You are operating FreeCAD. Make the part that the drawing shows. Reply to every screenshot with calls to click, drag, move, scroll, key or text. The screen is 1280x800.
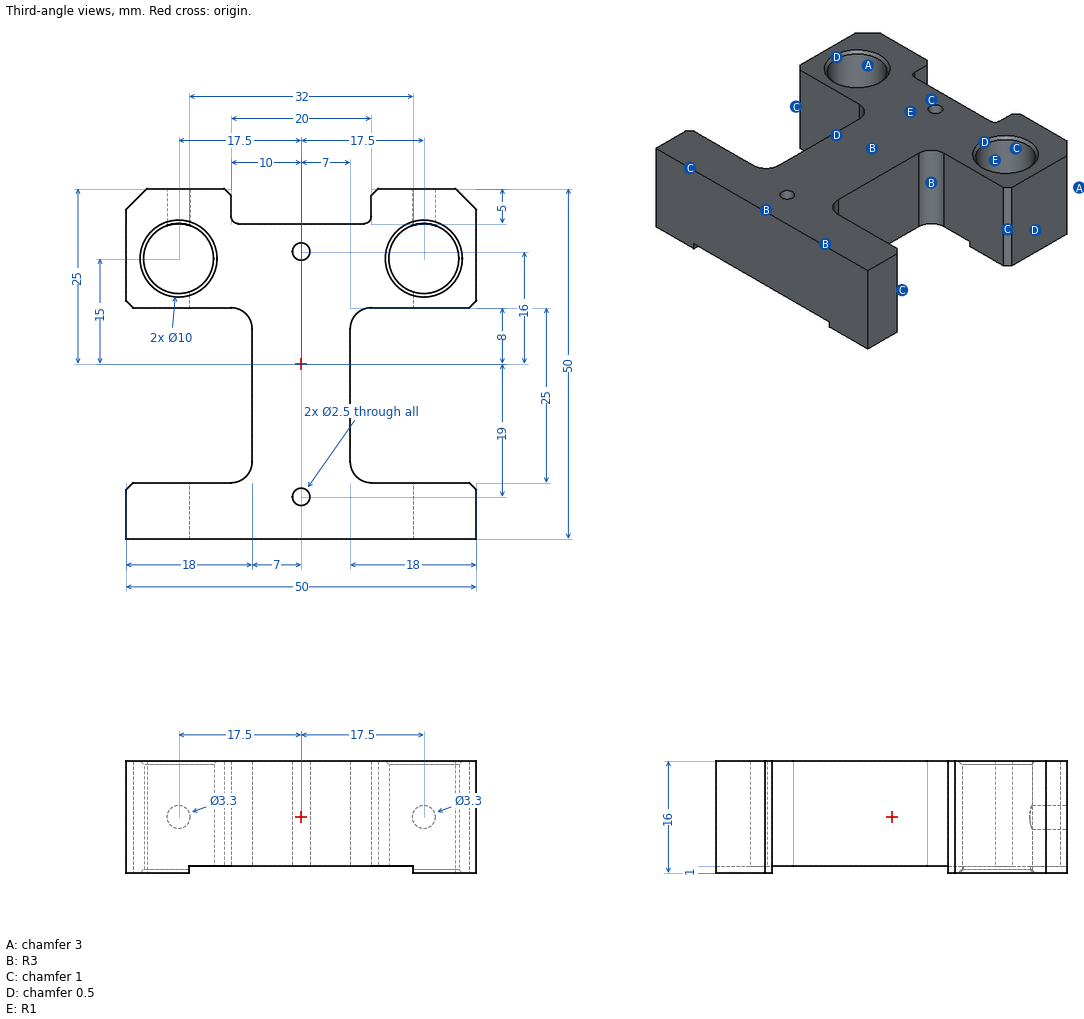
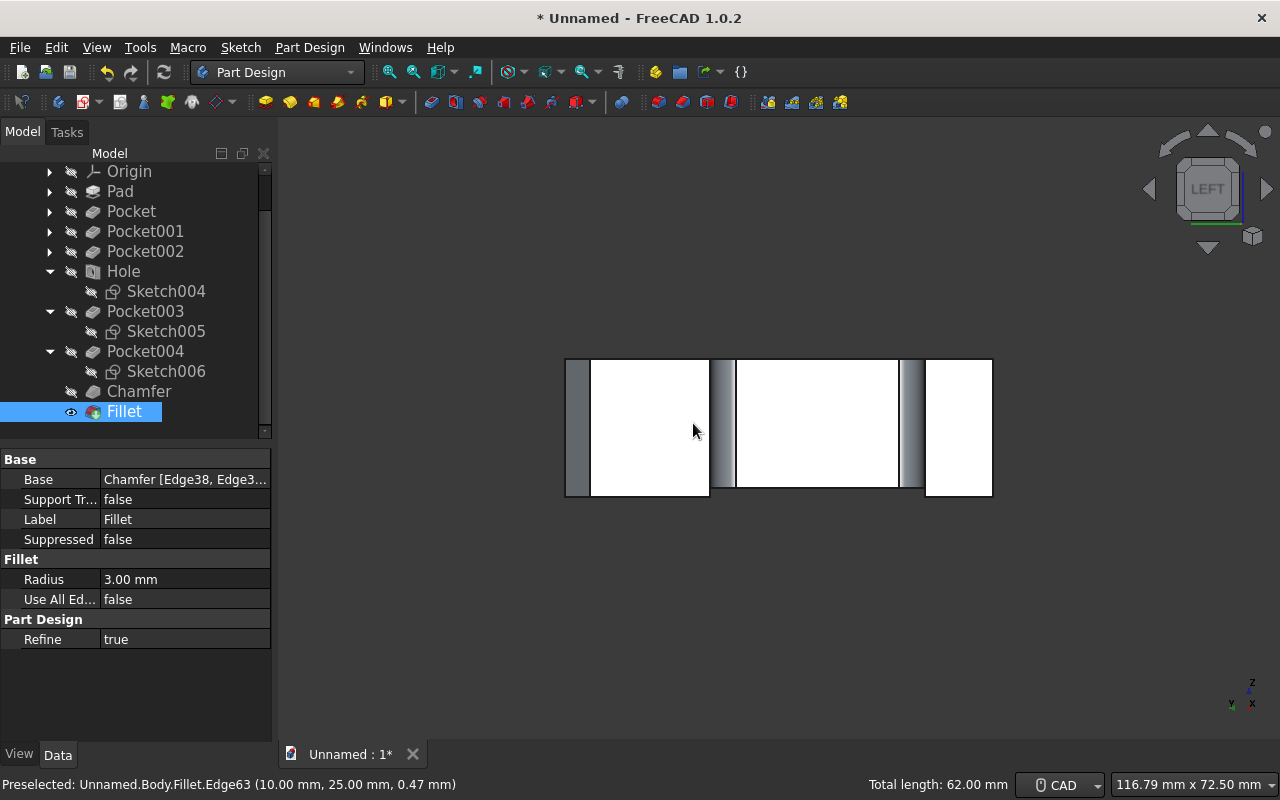
key(v)
key(f)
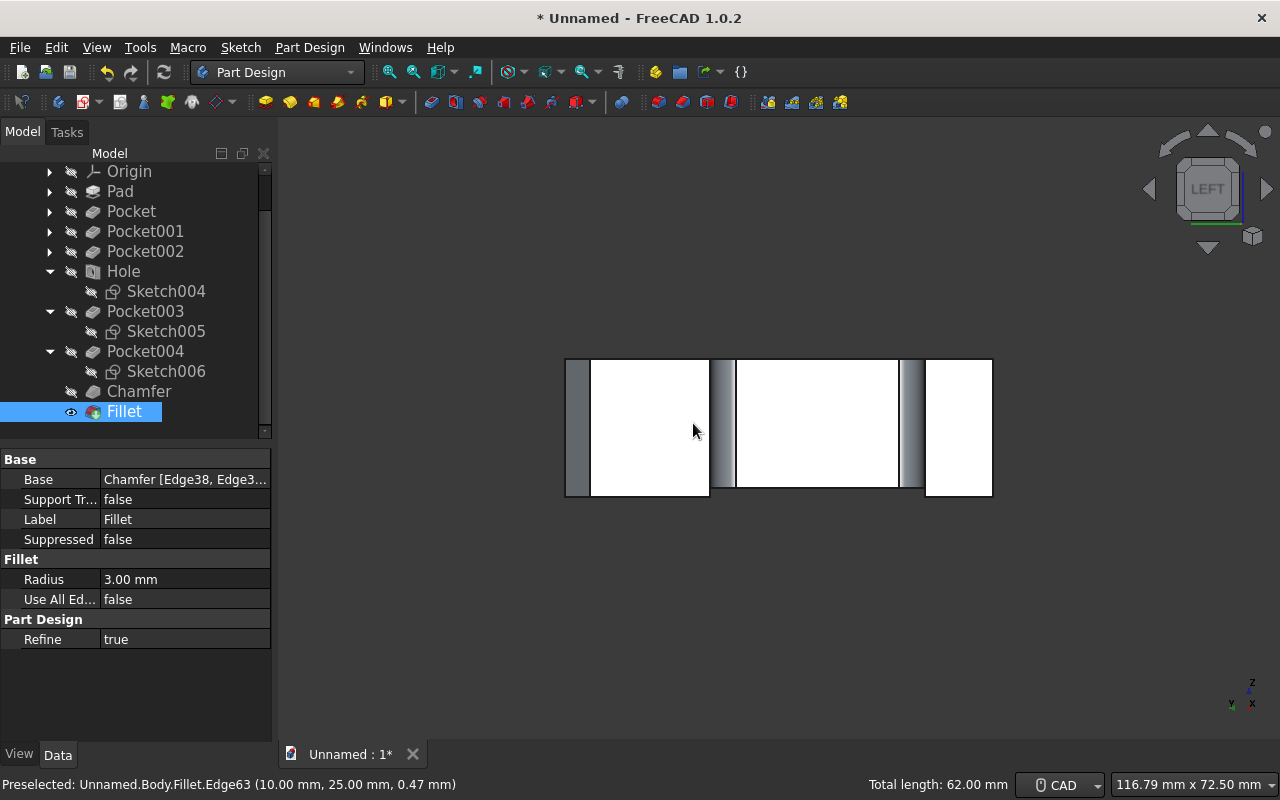
click(925, 427, ctrl)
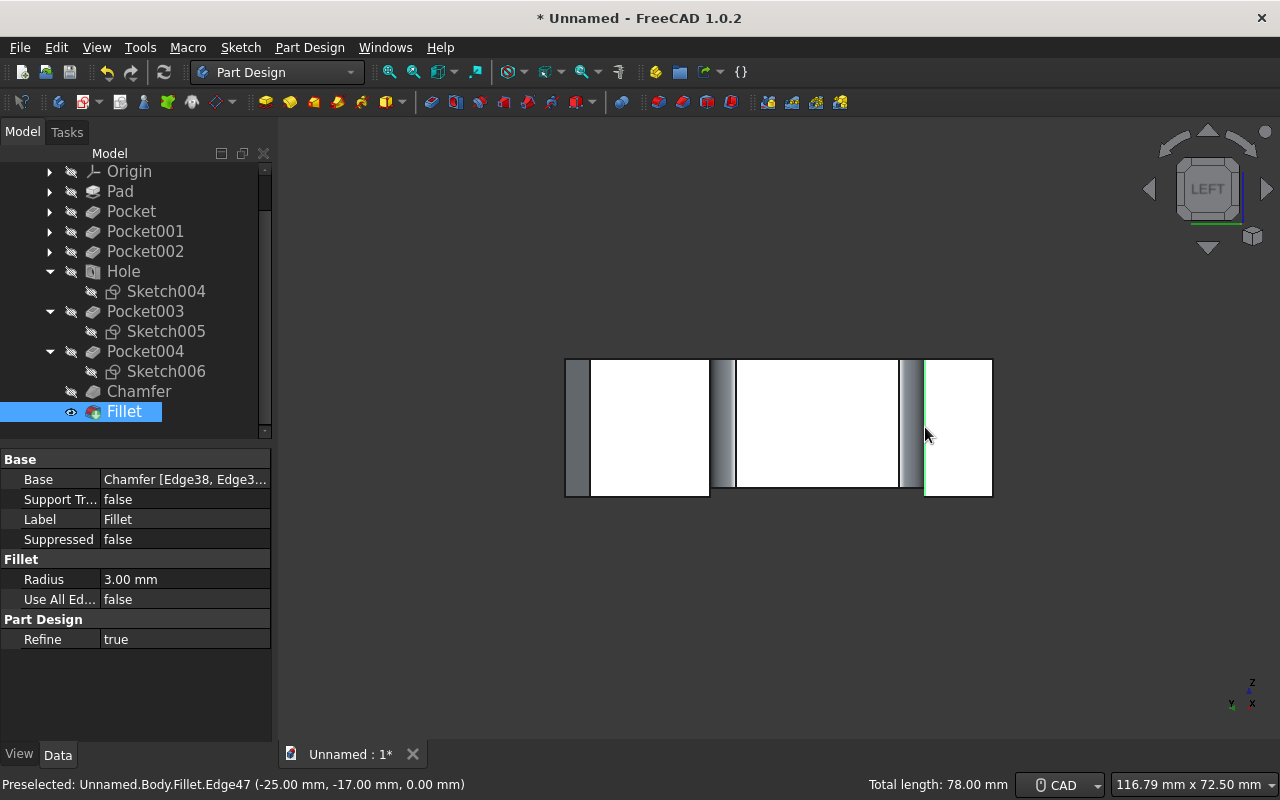
click(710, 427, ctrl)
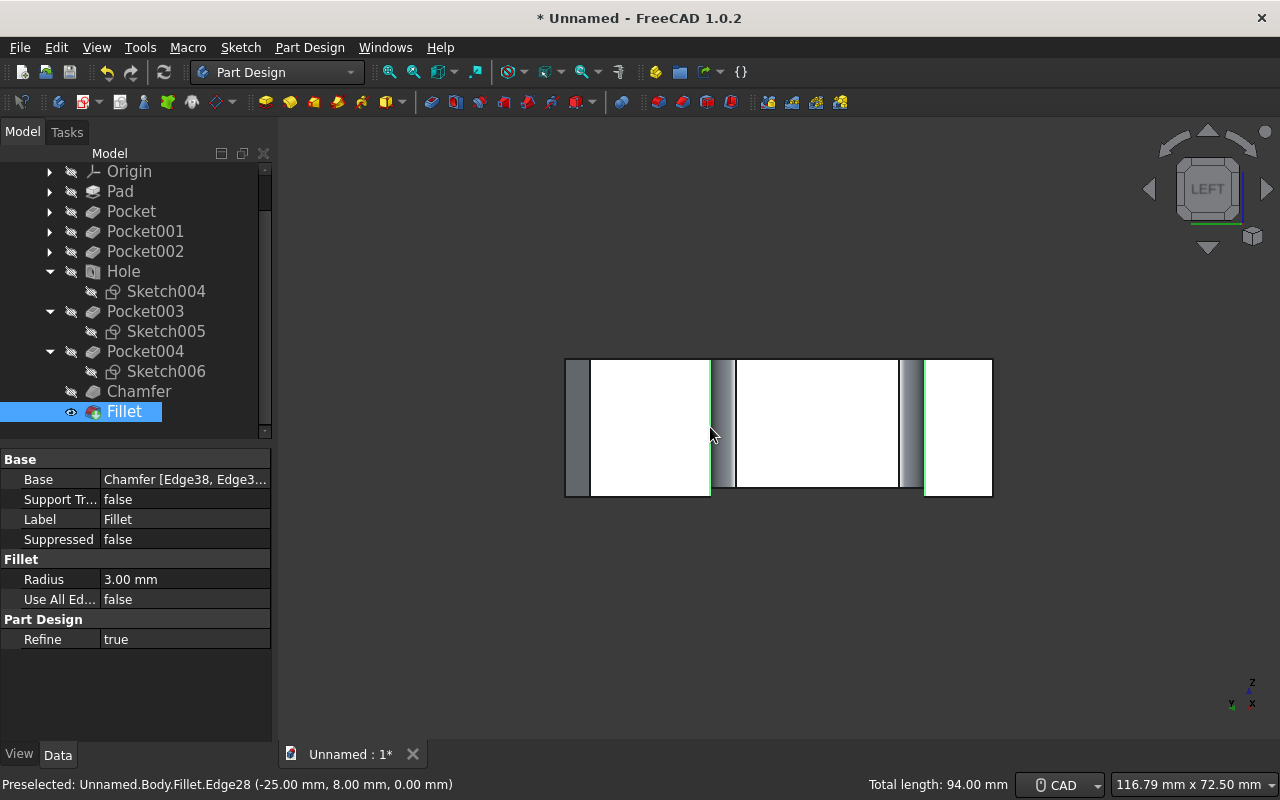
click(684, 102)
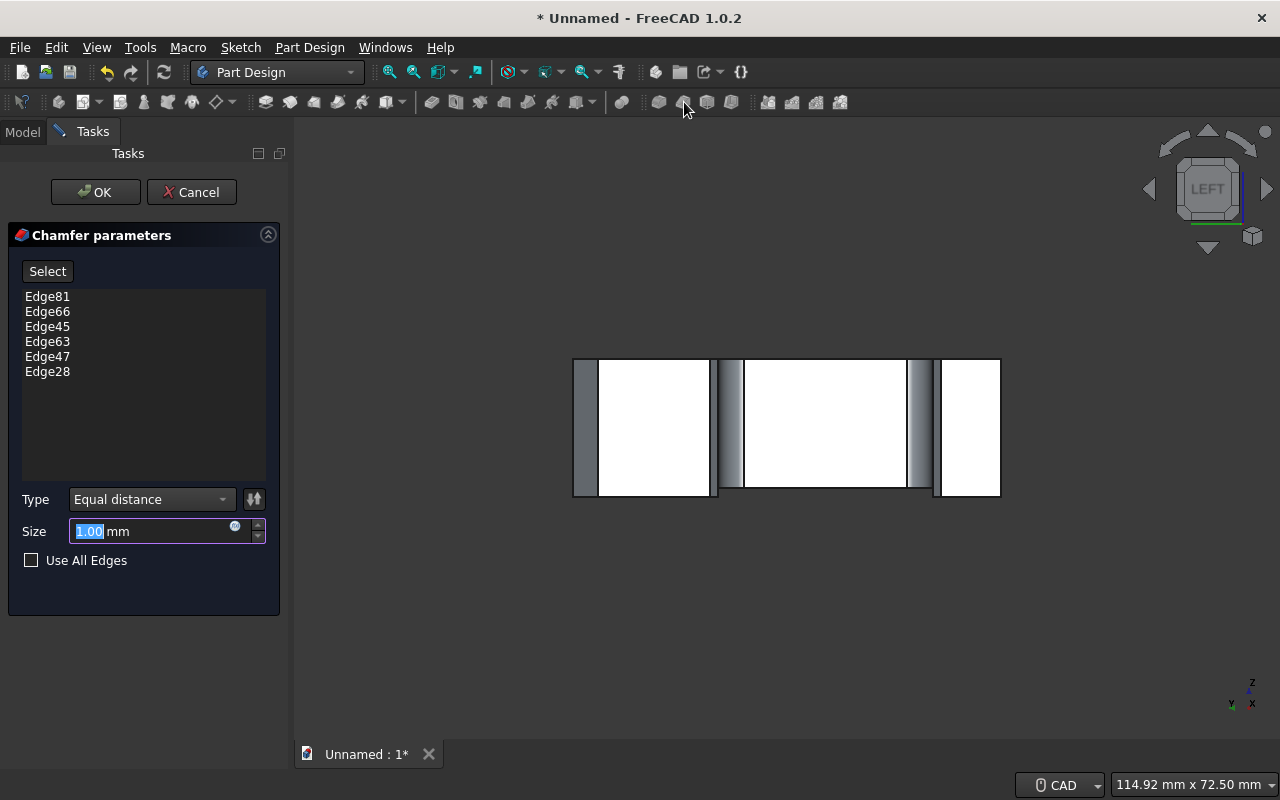
text(1)
key(Tab)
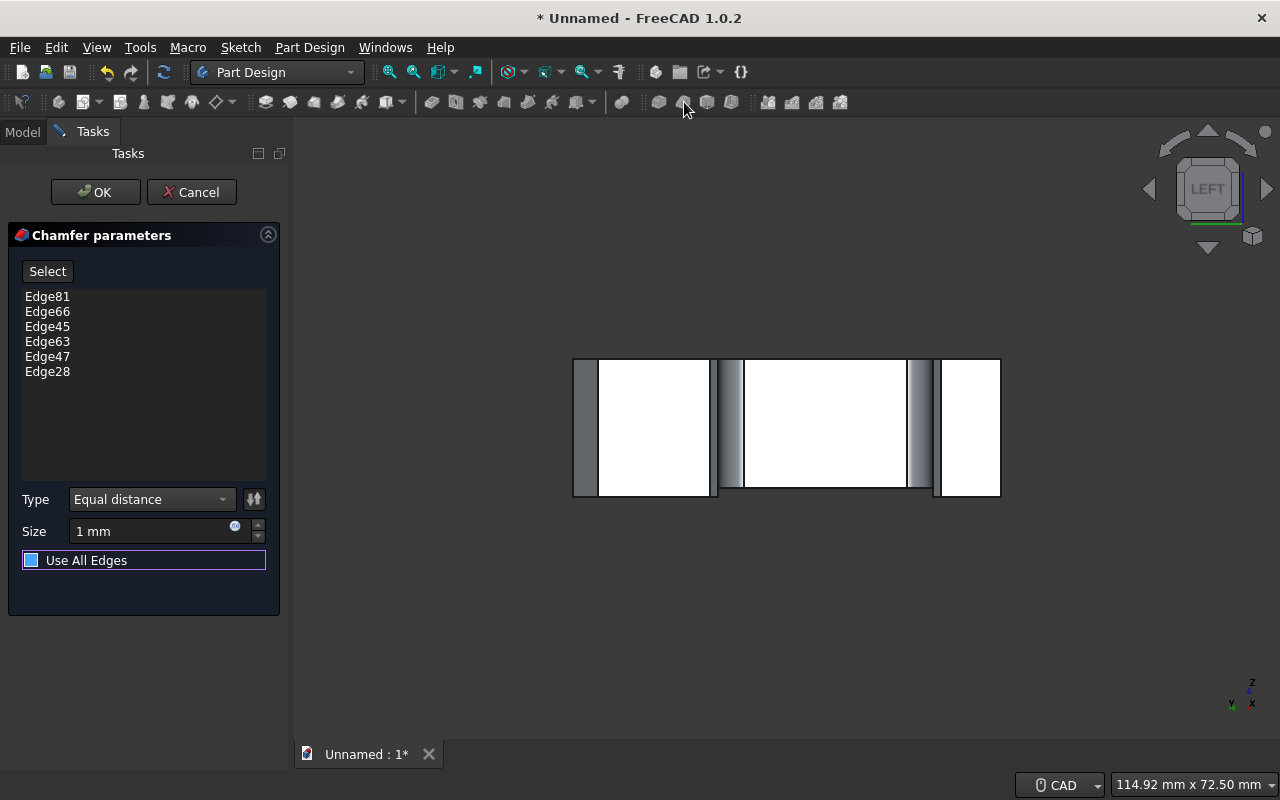
click(96, 192)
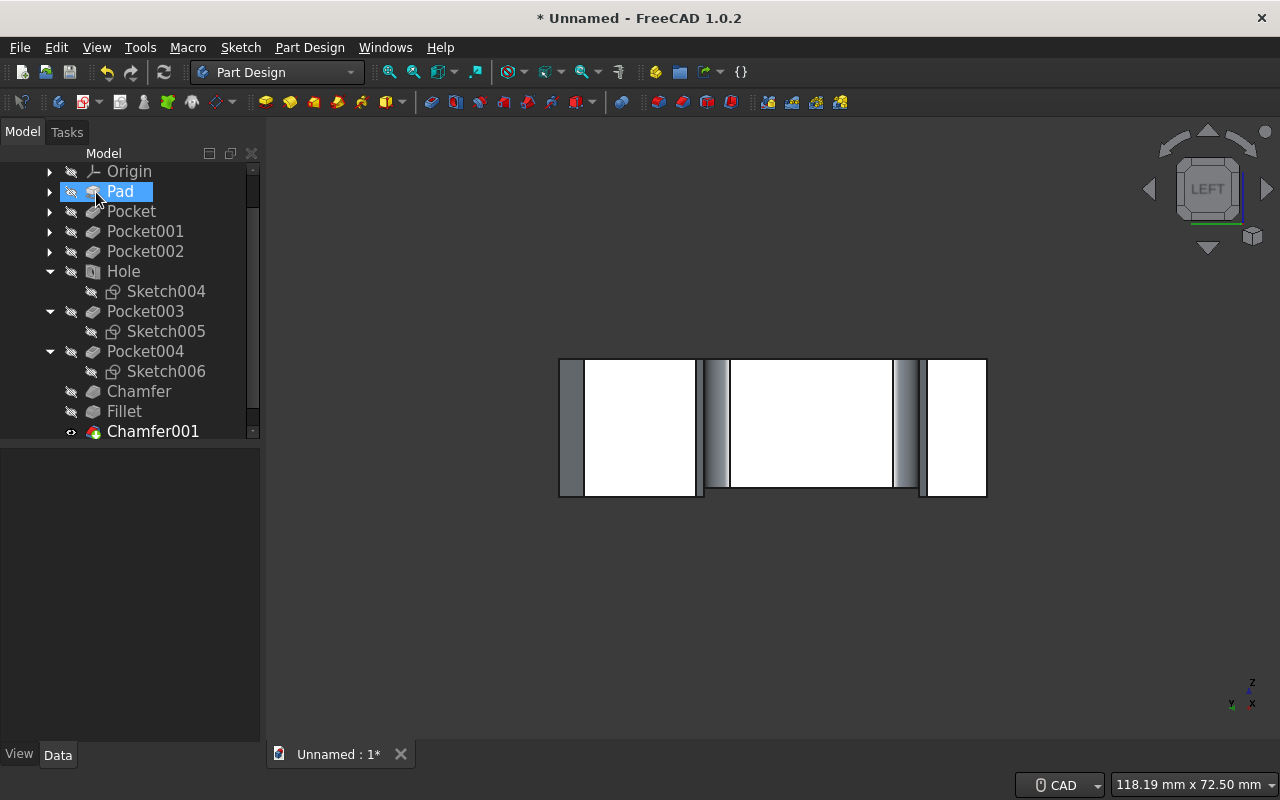
key(v)
key(f)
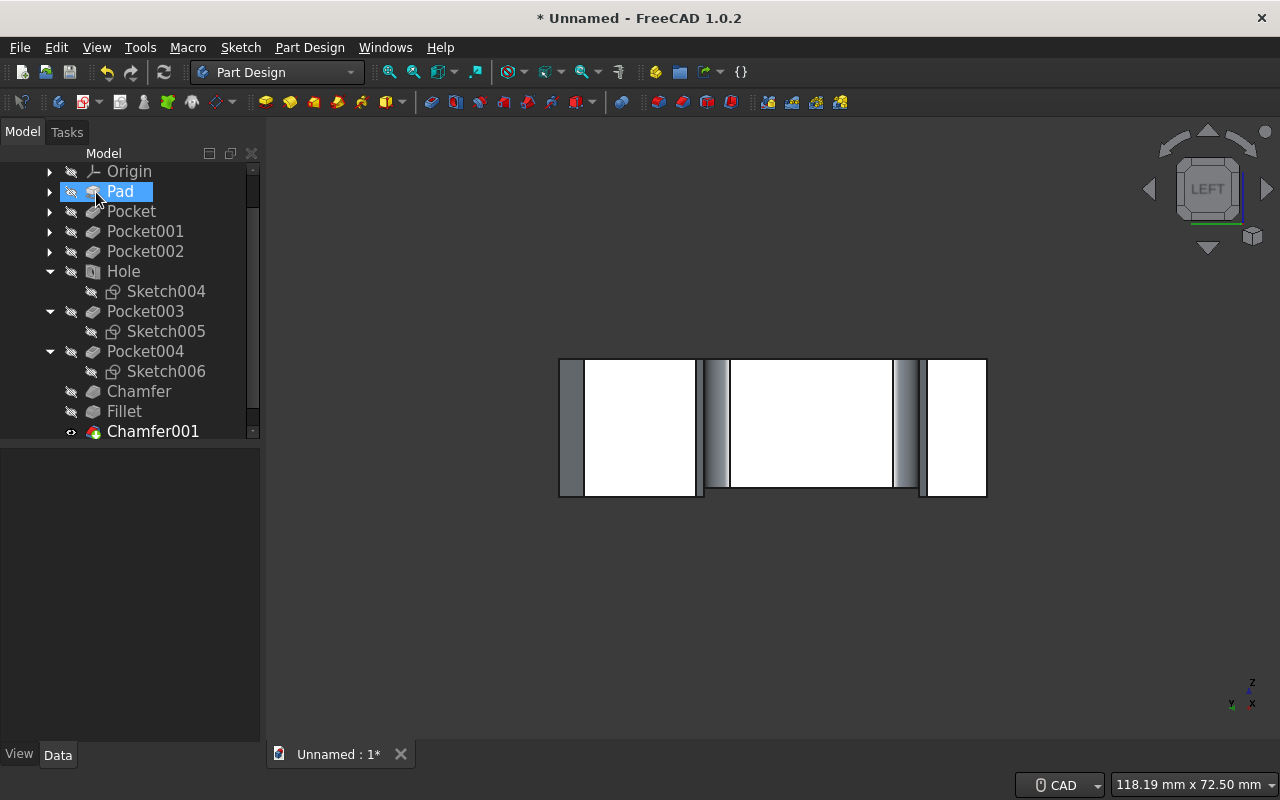
key(0)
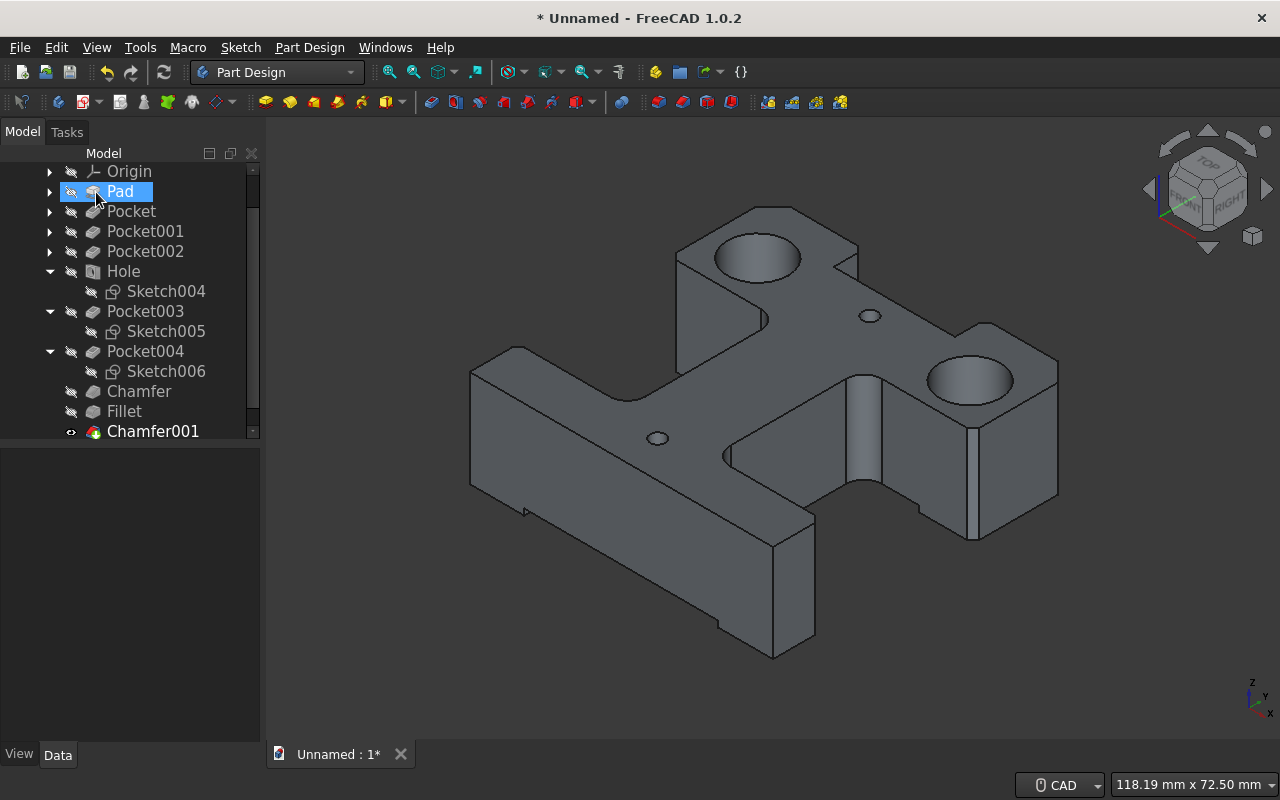
click(728, 240)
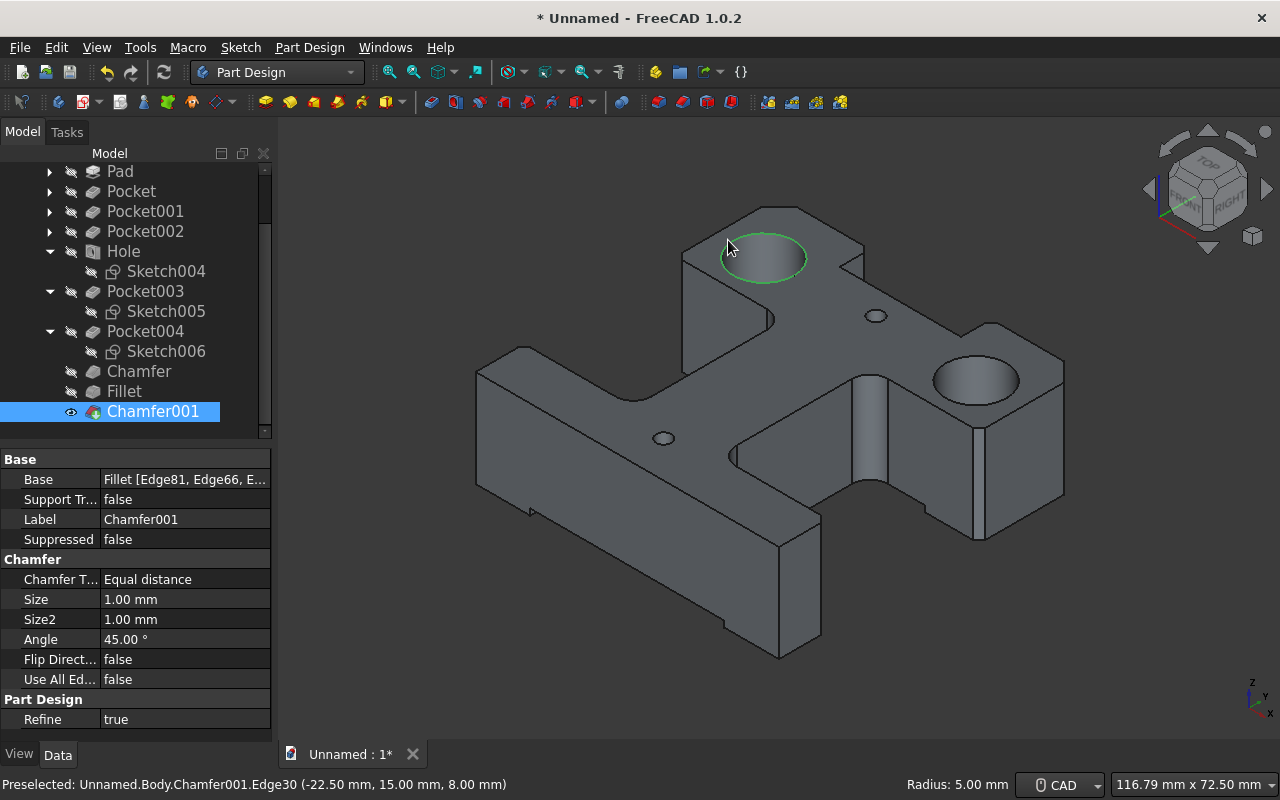
click(946, 362, ctrl)